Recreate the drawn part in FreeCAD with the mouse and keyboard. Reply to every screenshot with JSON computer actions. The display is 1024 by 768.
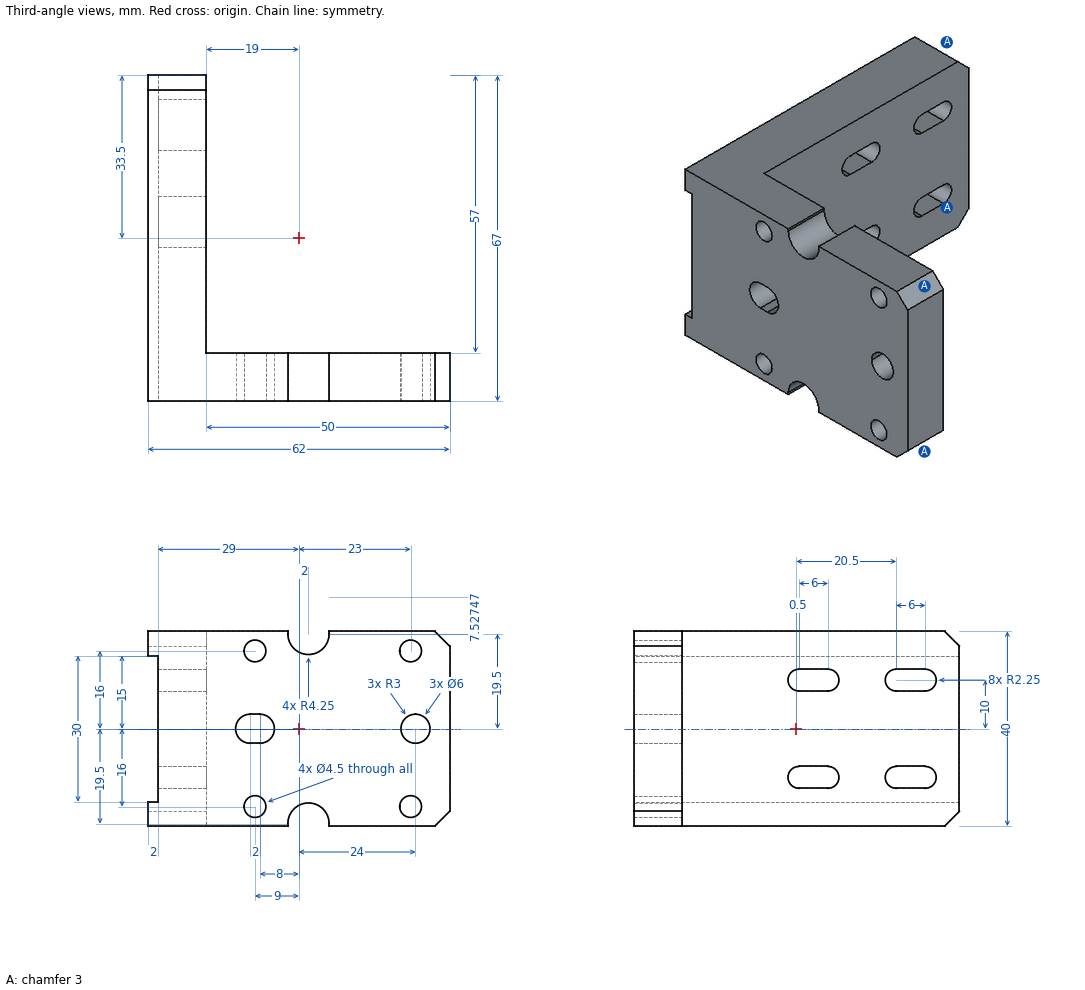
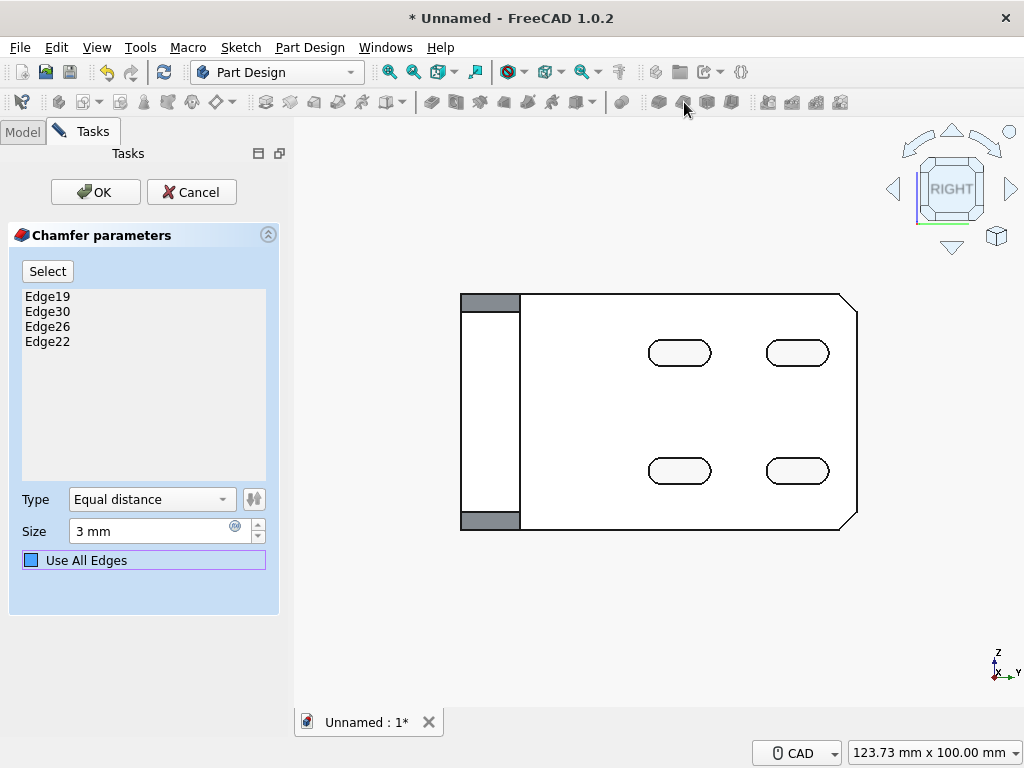
{"action": "left_click", "coordinate": [96, 192]}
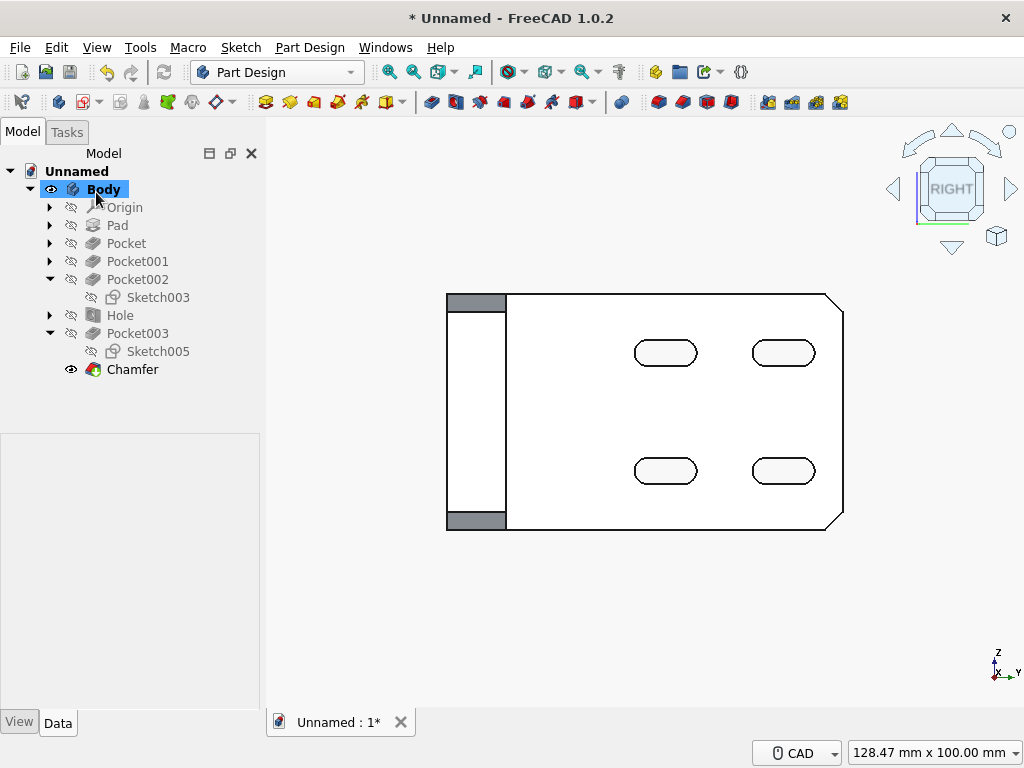
{"action": "key", "text": "4"}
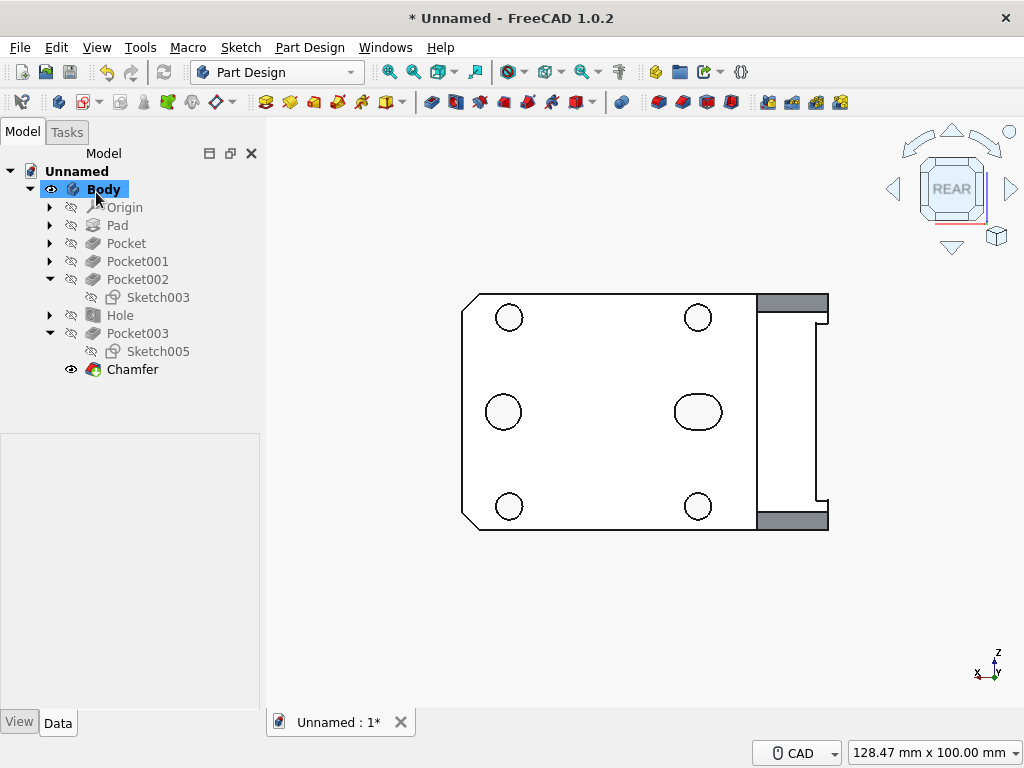
{"action": "left_click", "coordinate": [610, 377]}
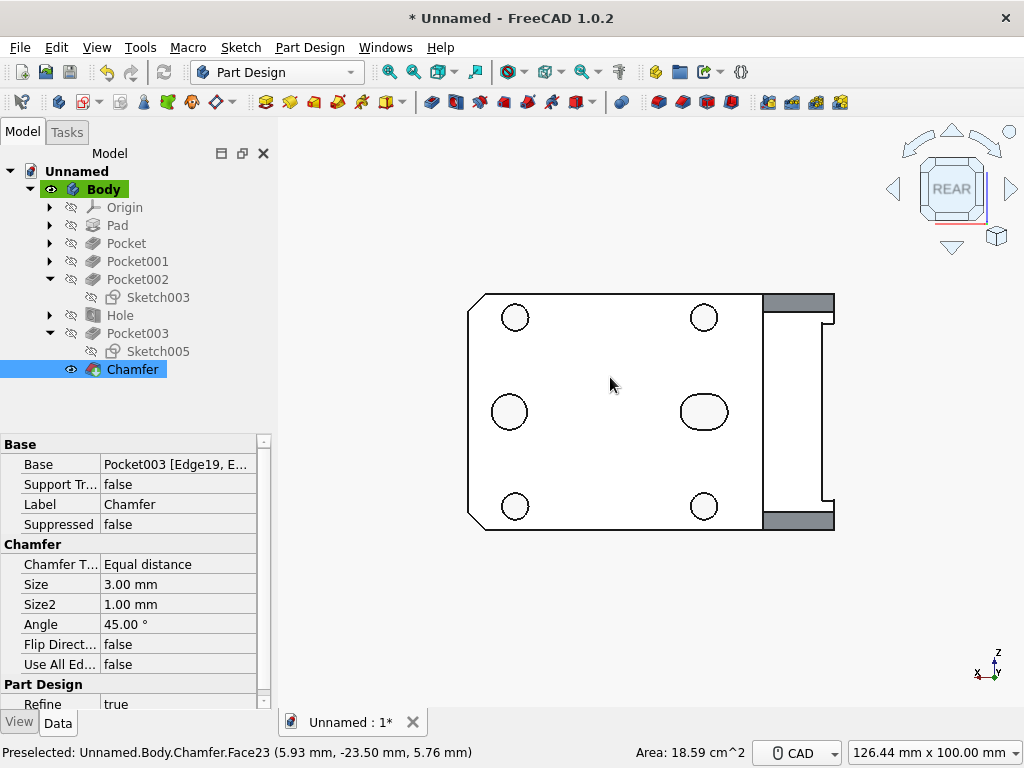
{"action": "left_click", "coordinate": [84, 102]}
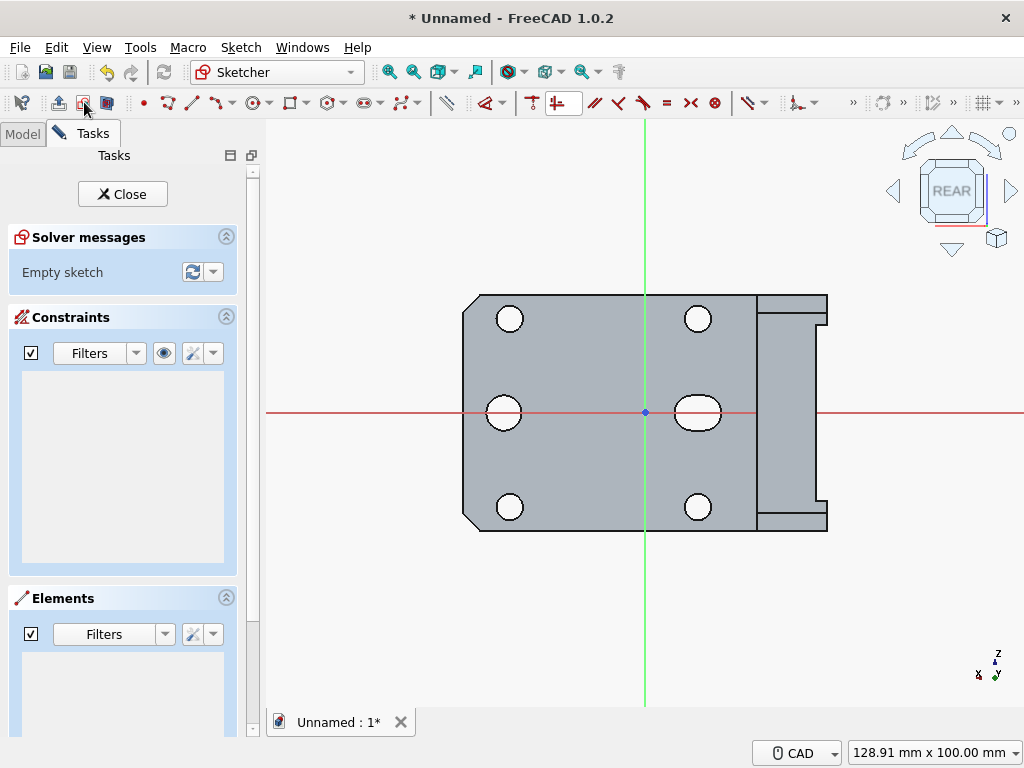
{"action": "left_click", "coordinate": [108, 104]}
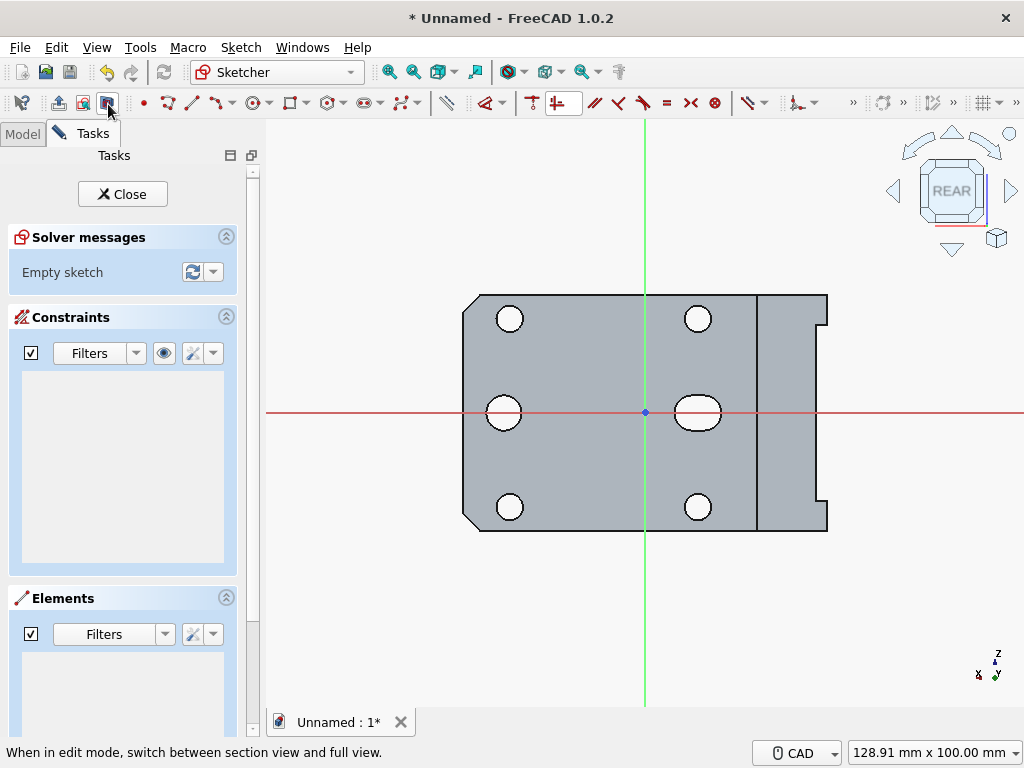
{"action": "left_click", "coordinate": [364, 104]}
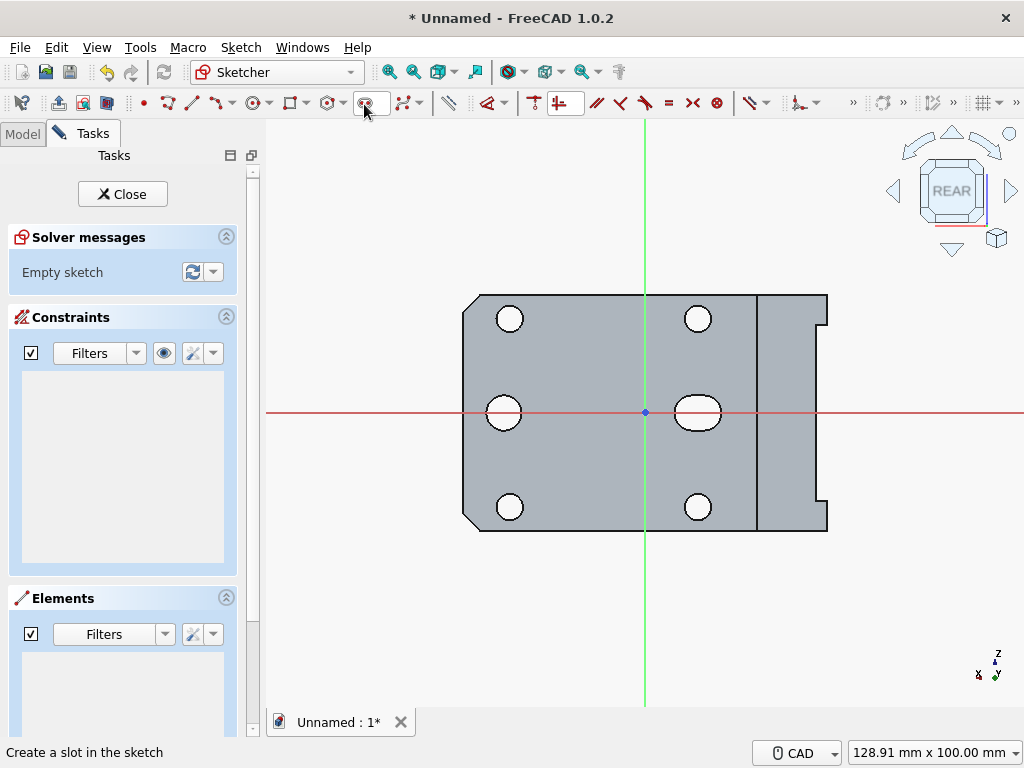
{"action": "scroll", "coordinate": [633, 298], "scroll_direction": "up", "scroll_amount": 2}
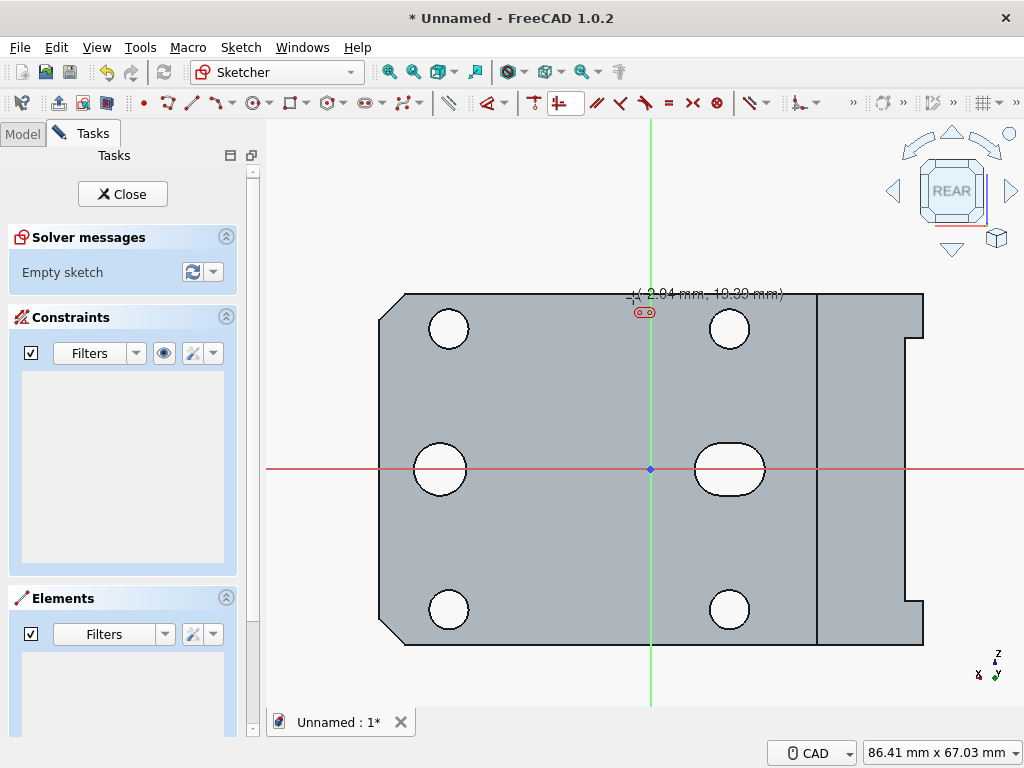
{"action": "left_click", "coordinate": [633, 298]}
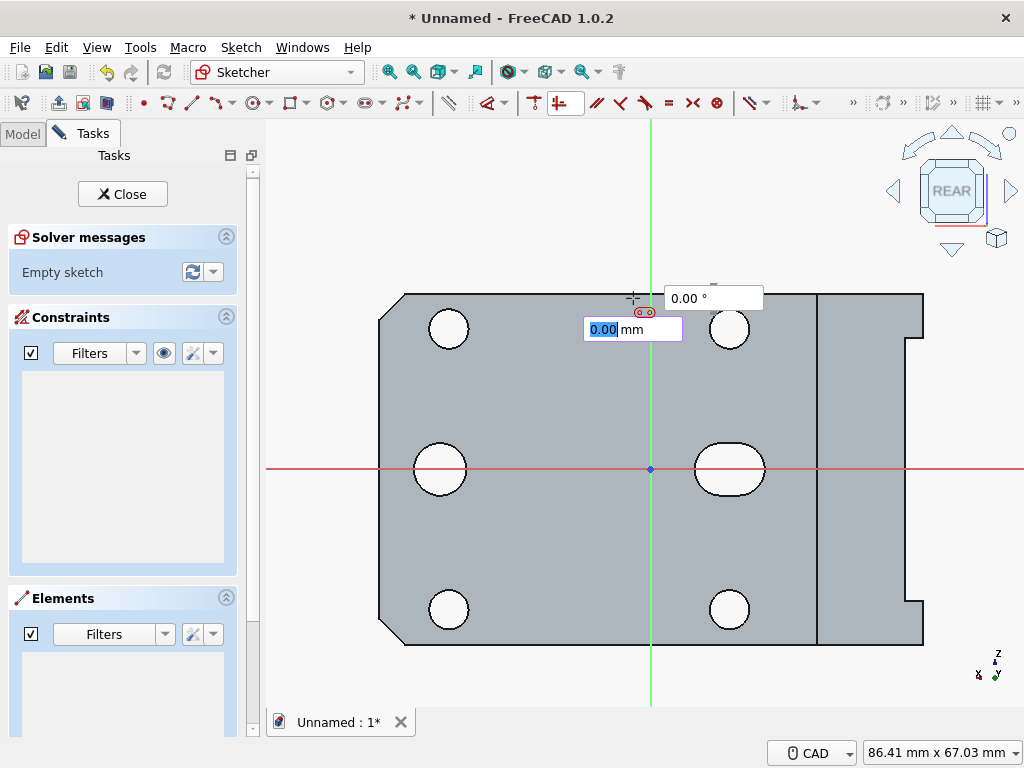
{"action": "left_click", "coordinate": [633, 232]}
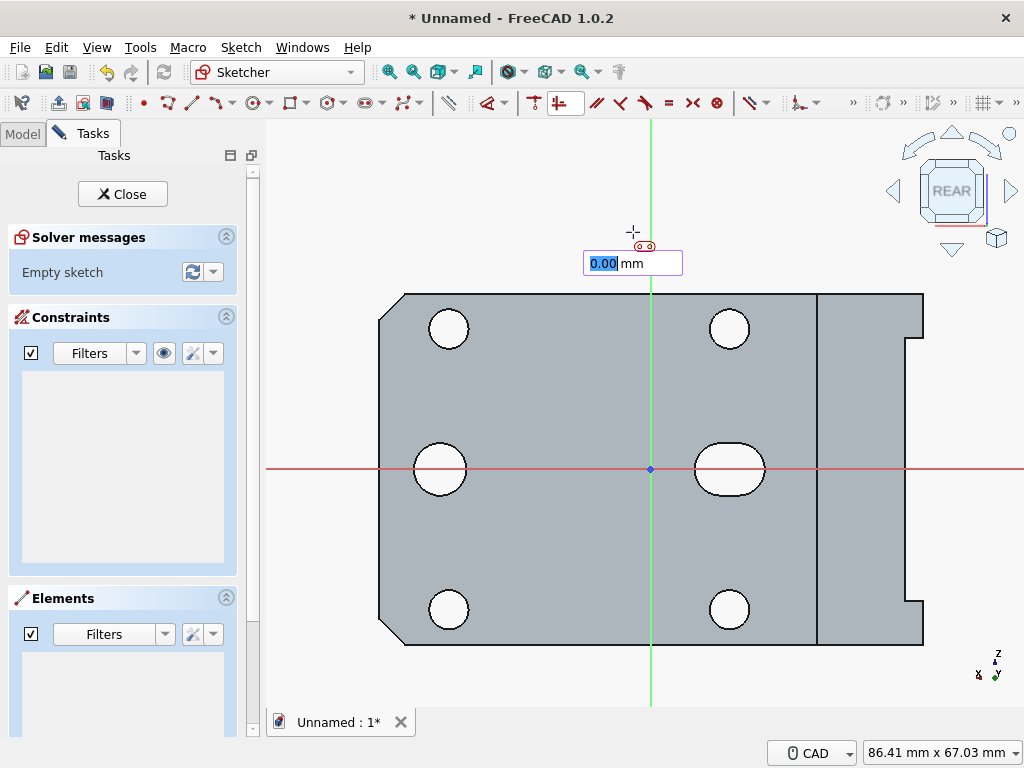
{"action": "left_click", "coordinate": [596, 265]}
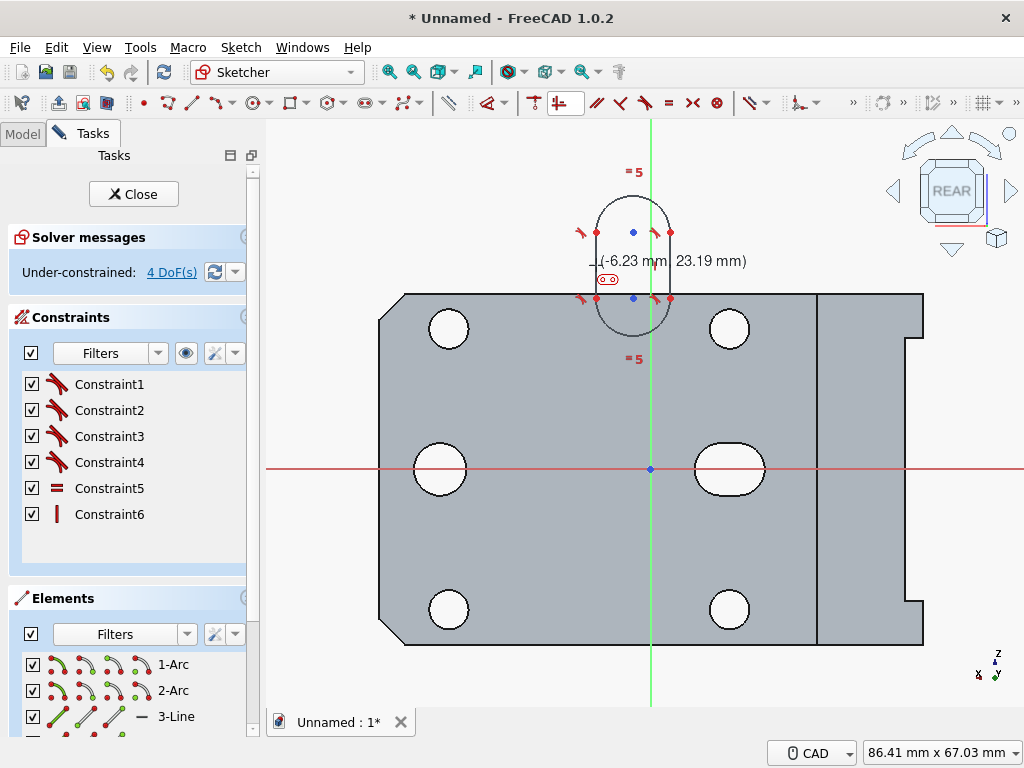
{"action": "scroll", "coordinate": [461, 298], "scroll_direction": "down", "scroll_amount": 2}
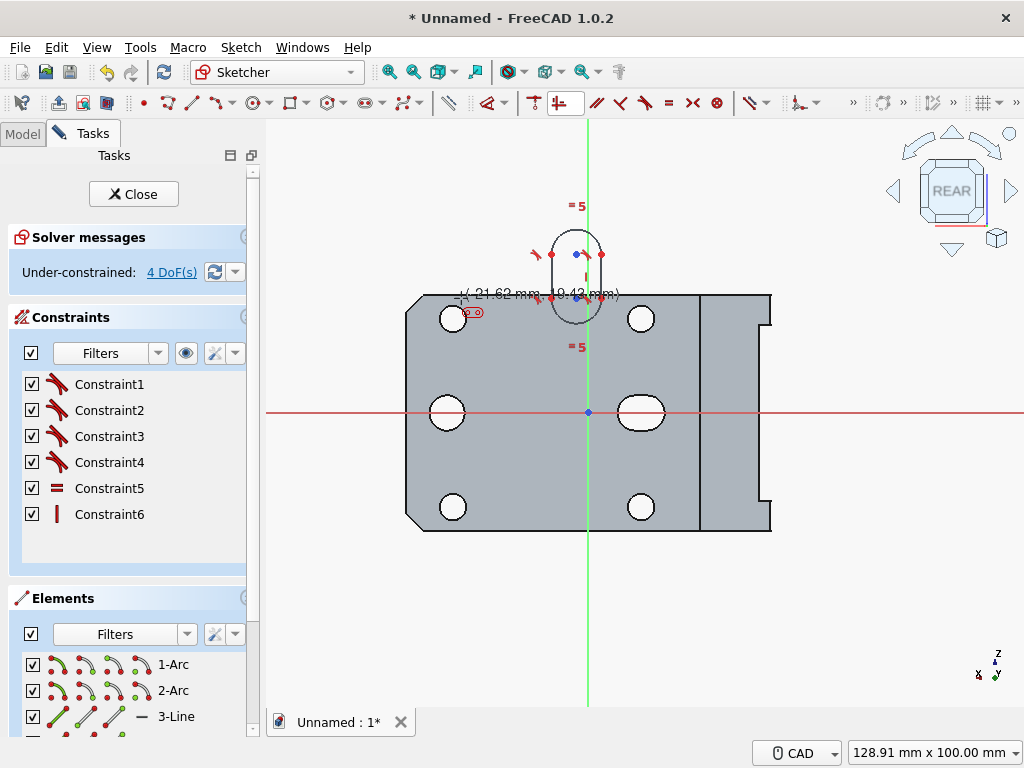
{"action": "scroll", "coordinate": [576, 572], "scroll_direction": "up", "scroll_amount": 2}